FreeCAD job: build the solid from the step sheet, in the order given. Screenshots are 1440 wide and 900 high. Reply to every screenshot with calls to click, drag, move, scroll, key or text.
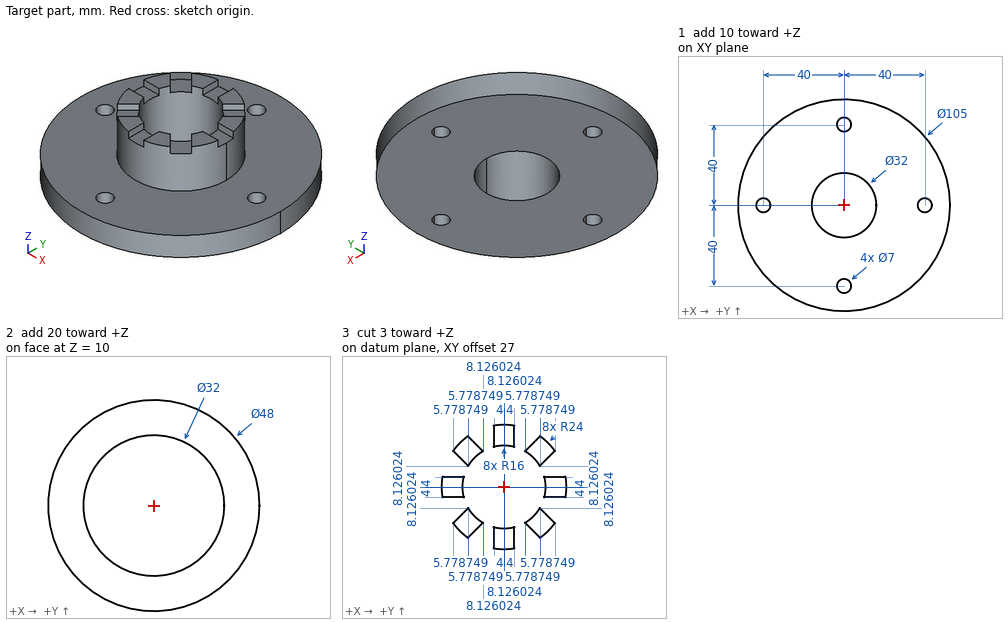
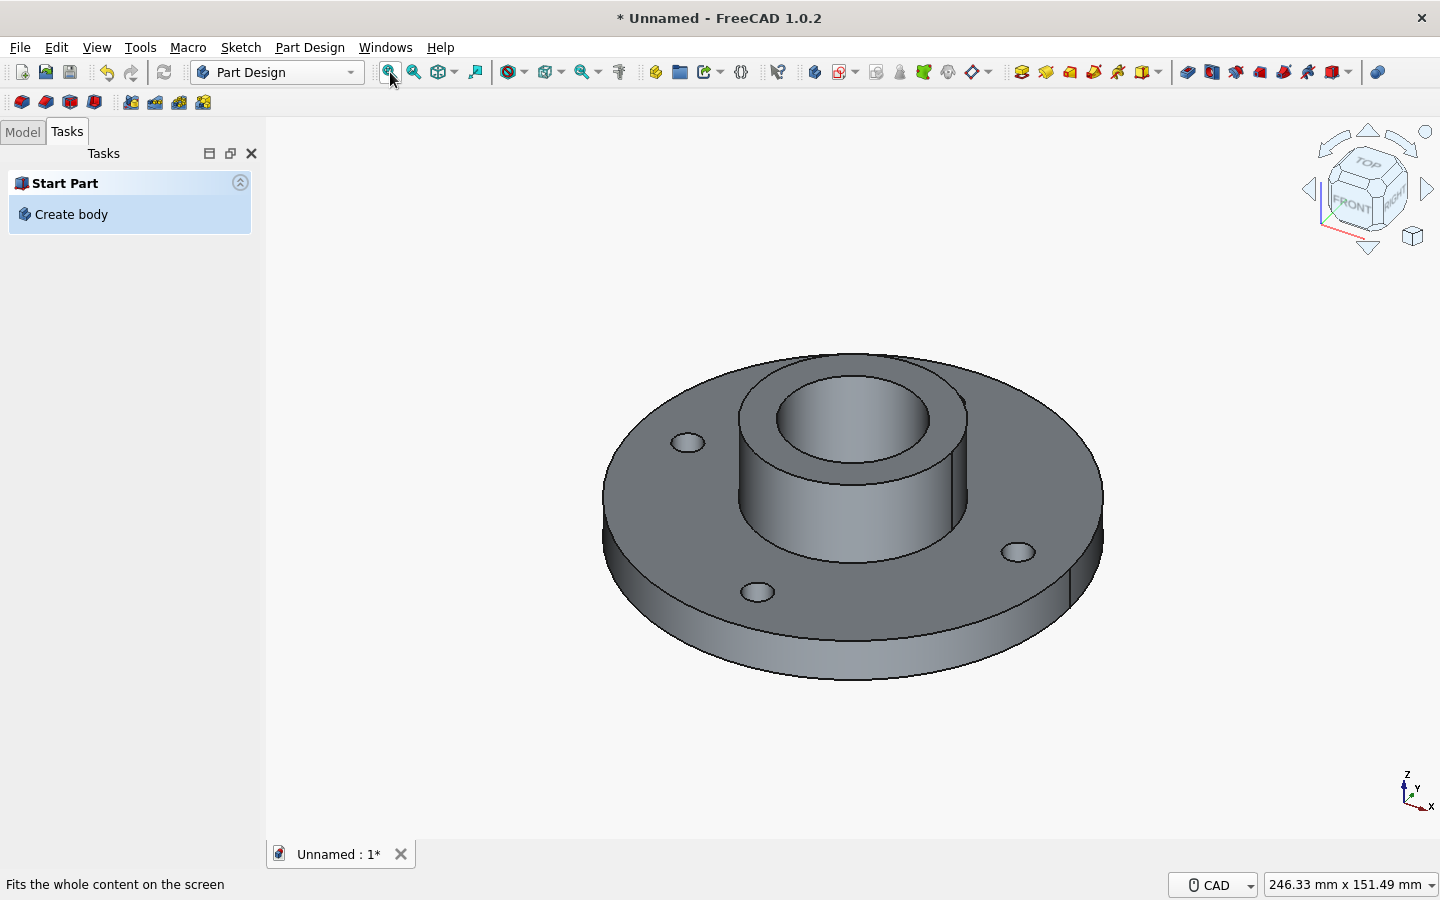
click(23, 131)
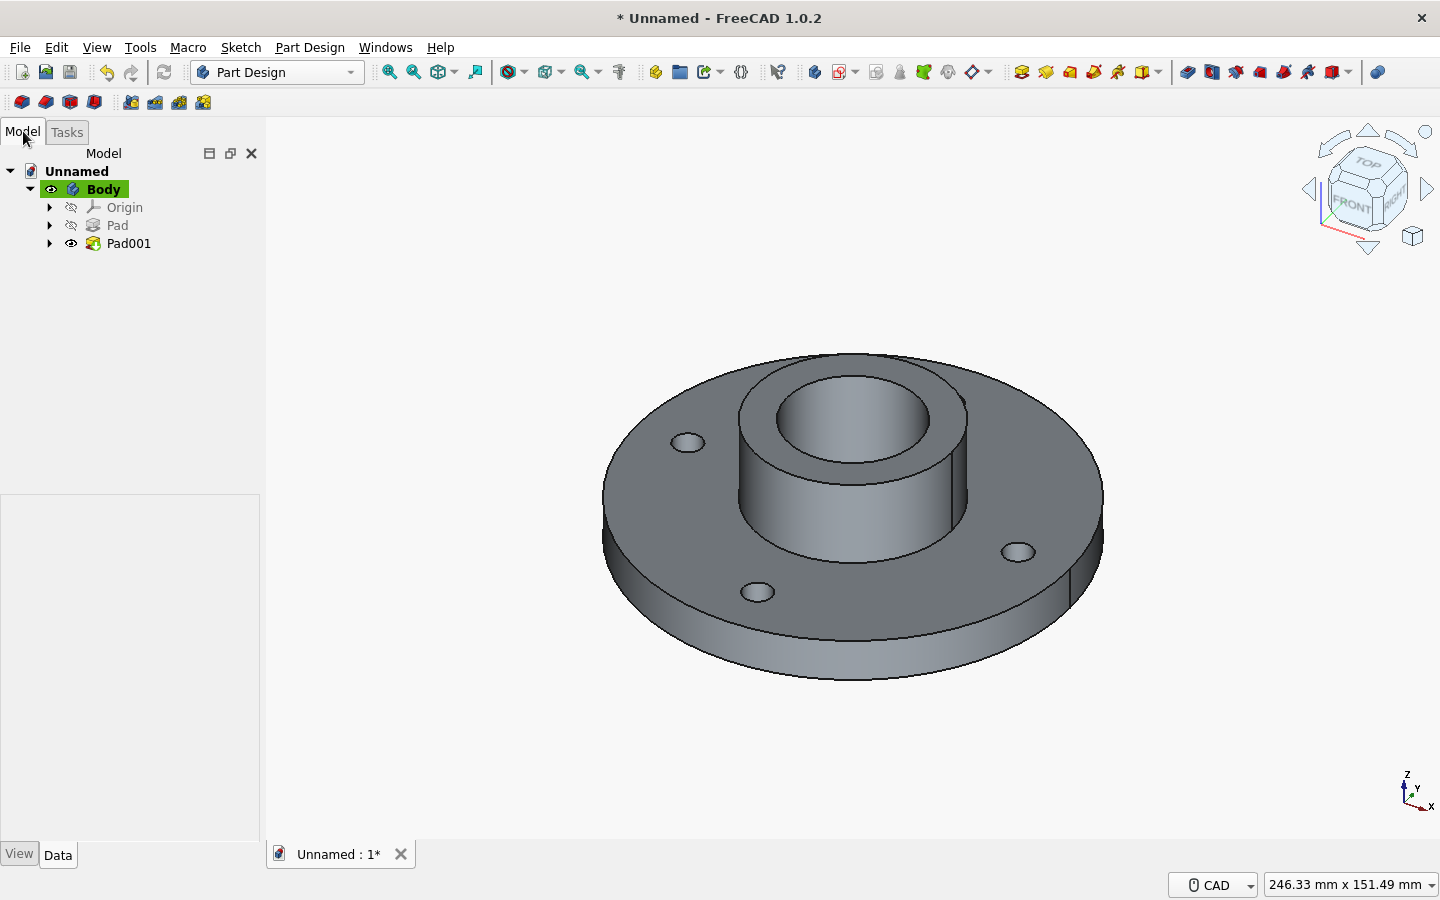
click(50, 207)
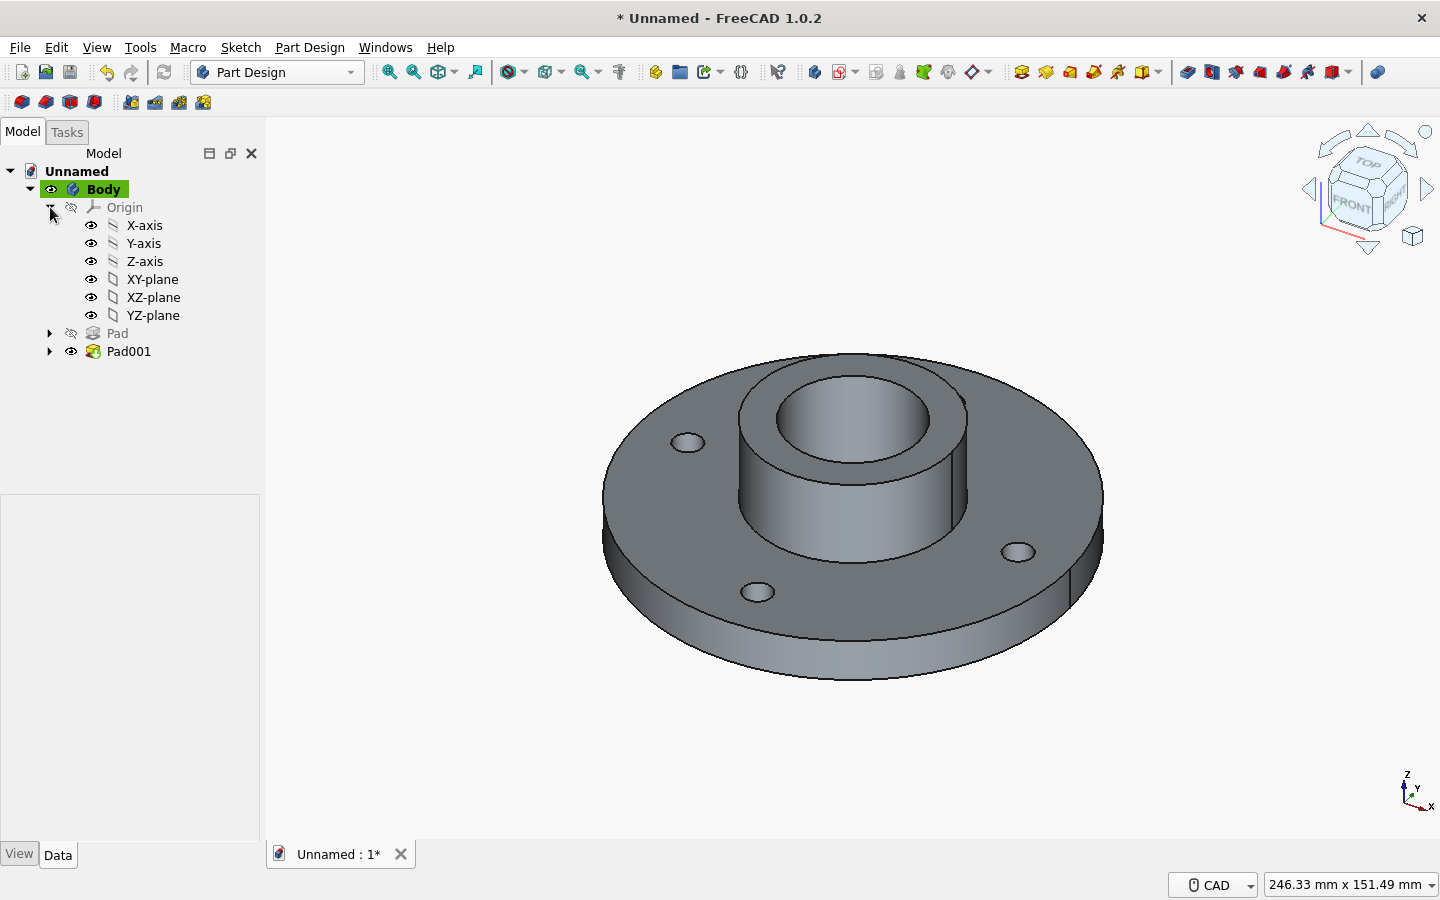
click(136, 279)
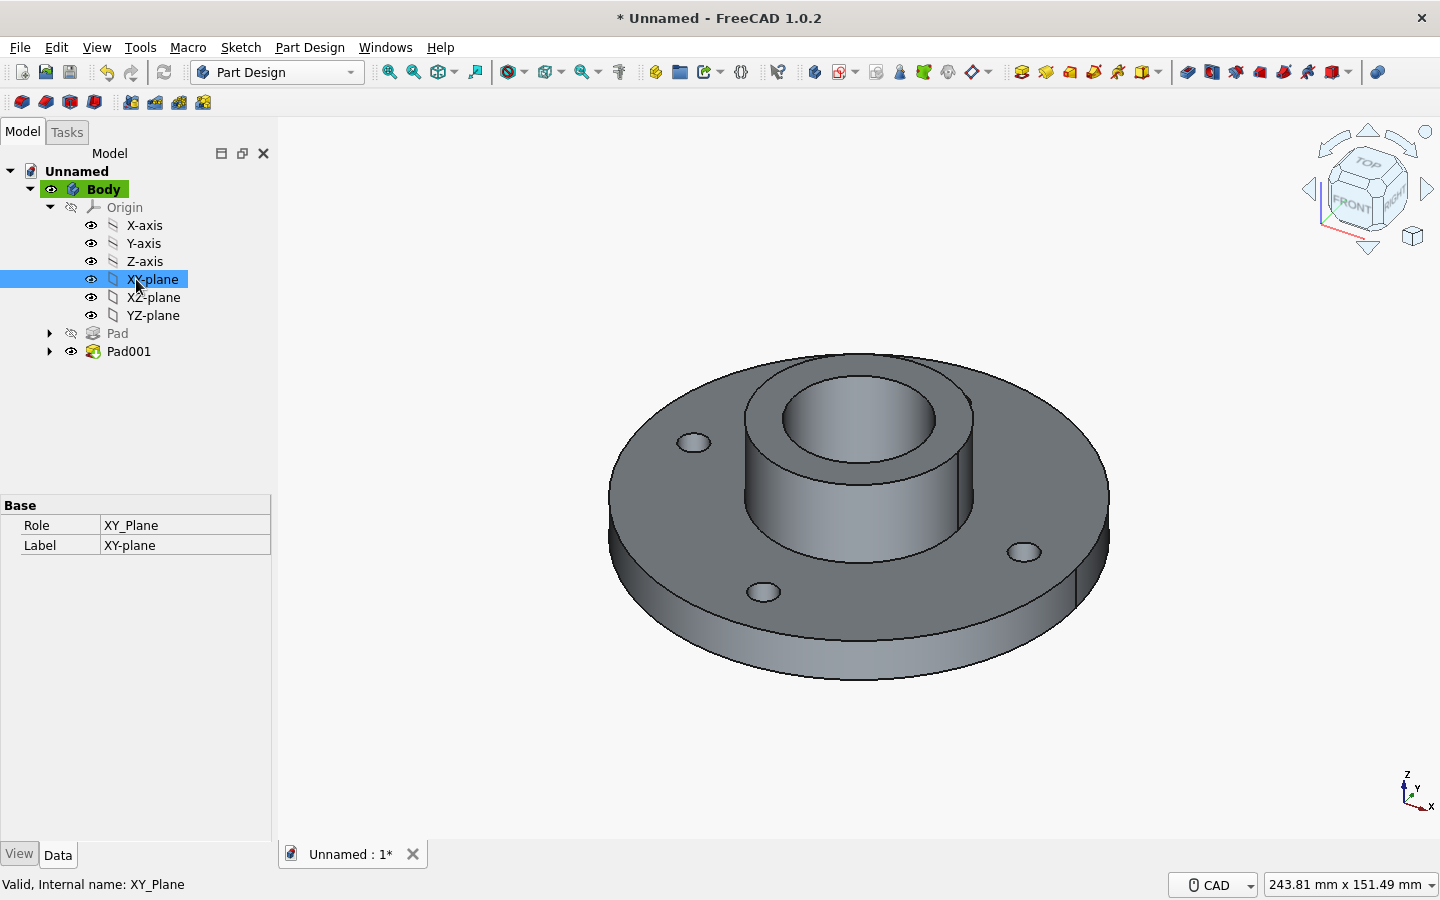
click(972, 72)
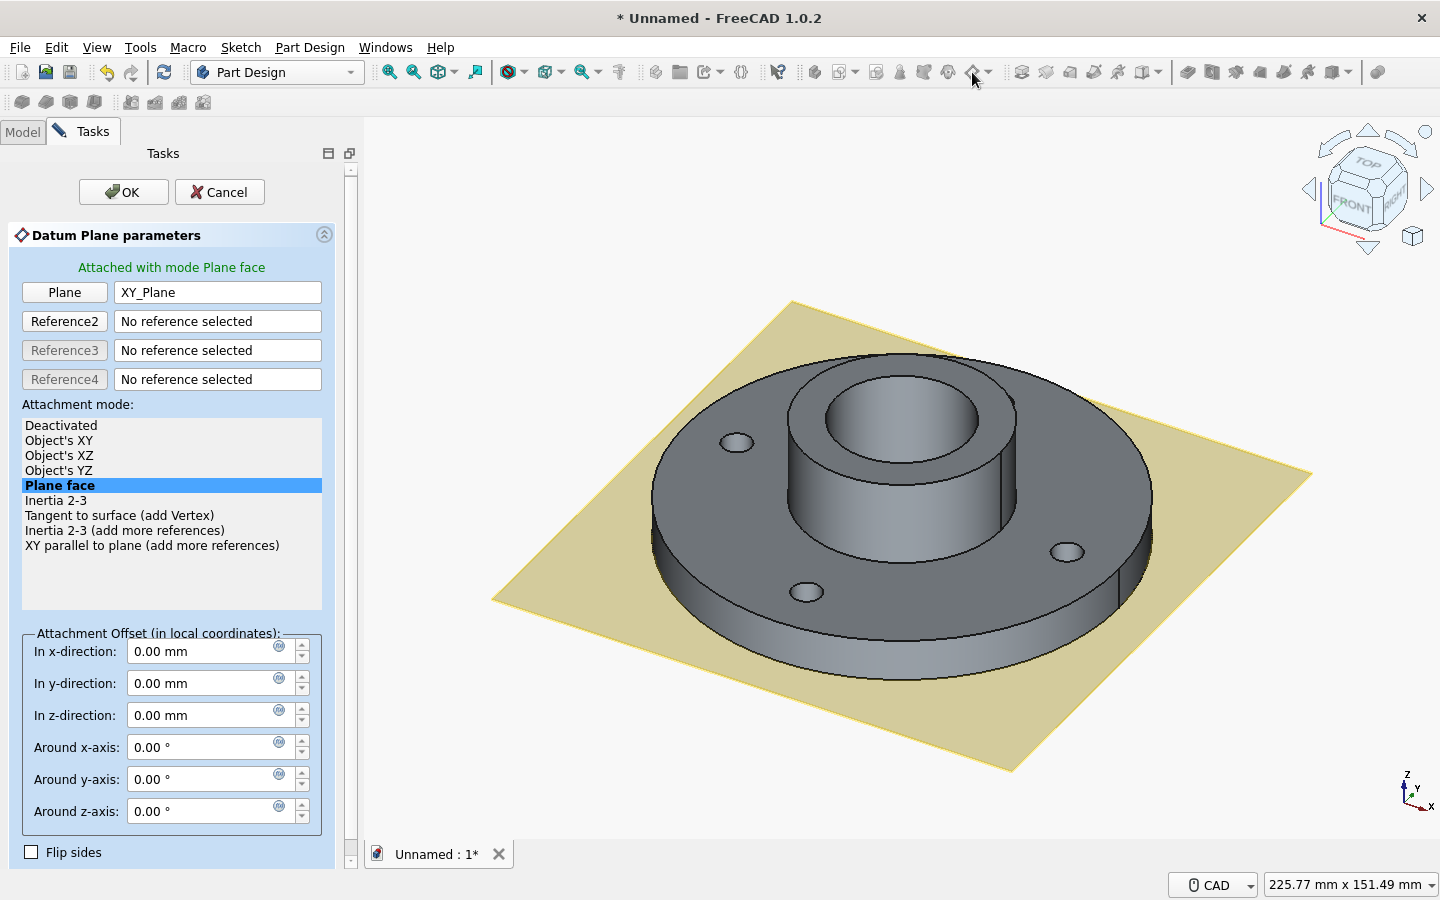
triple_click(210, 715)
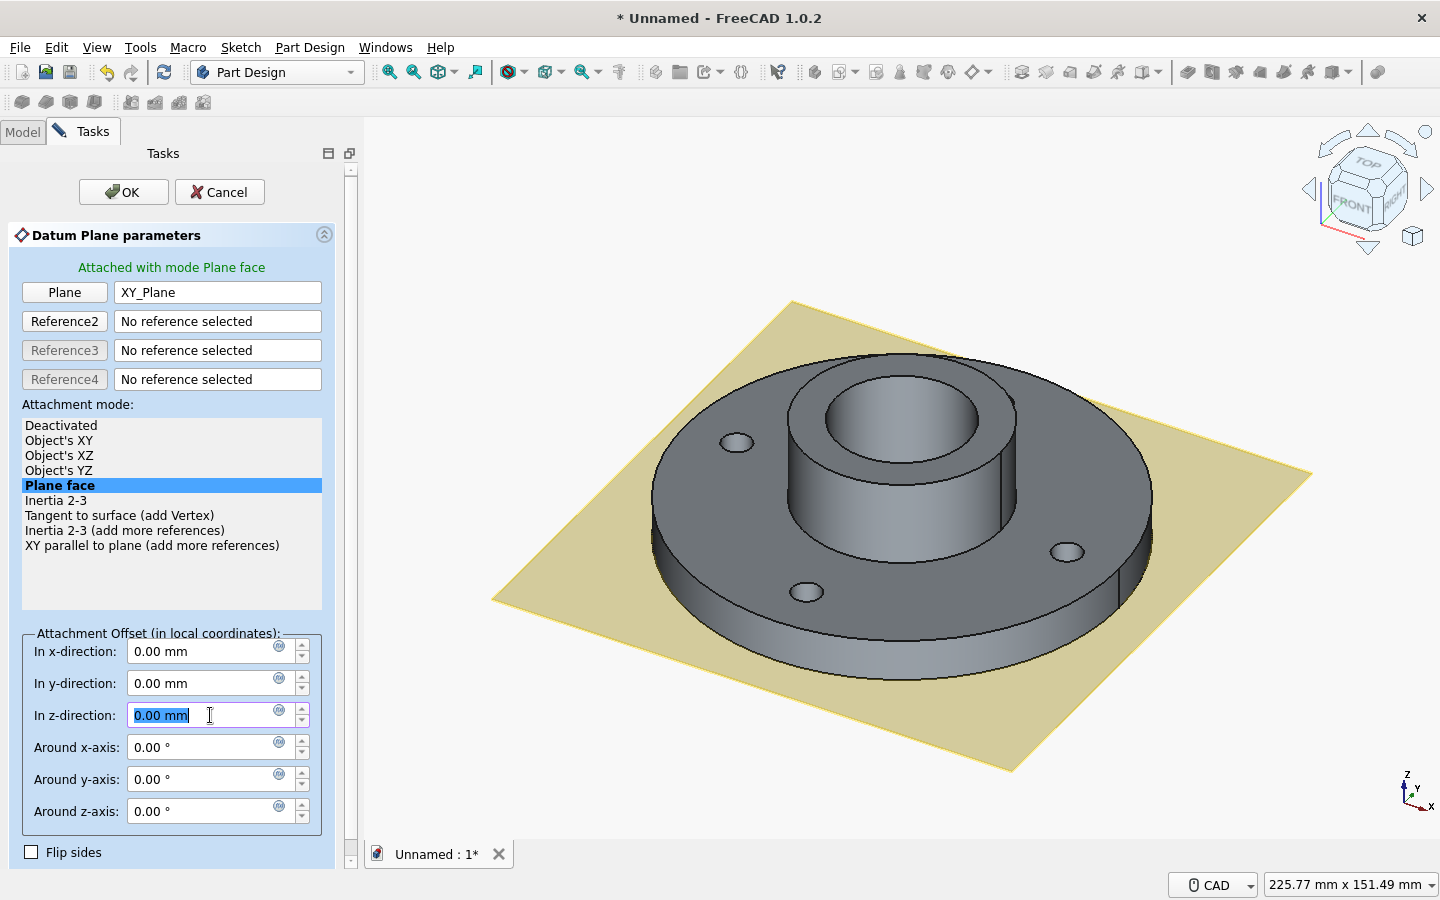
text(27)
key(Tab)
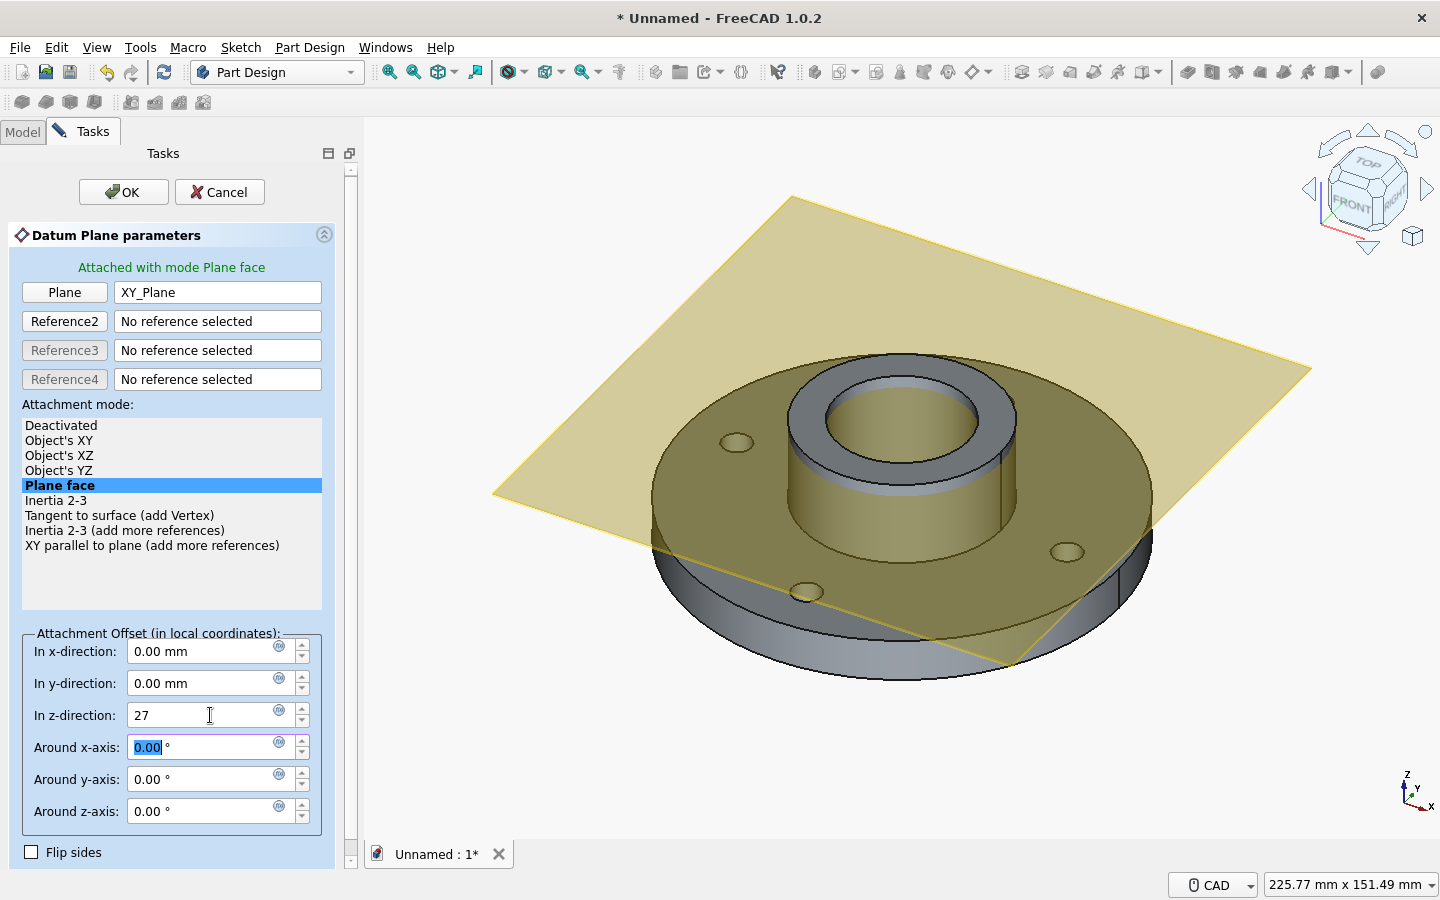
click(124, 192)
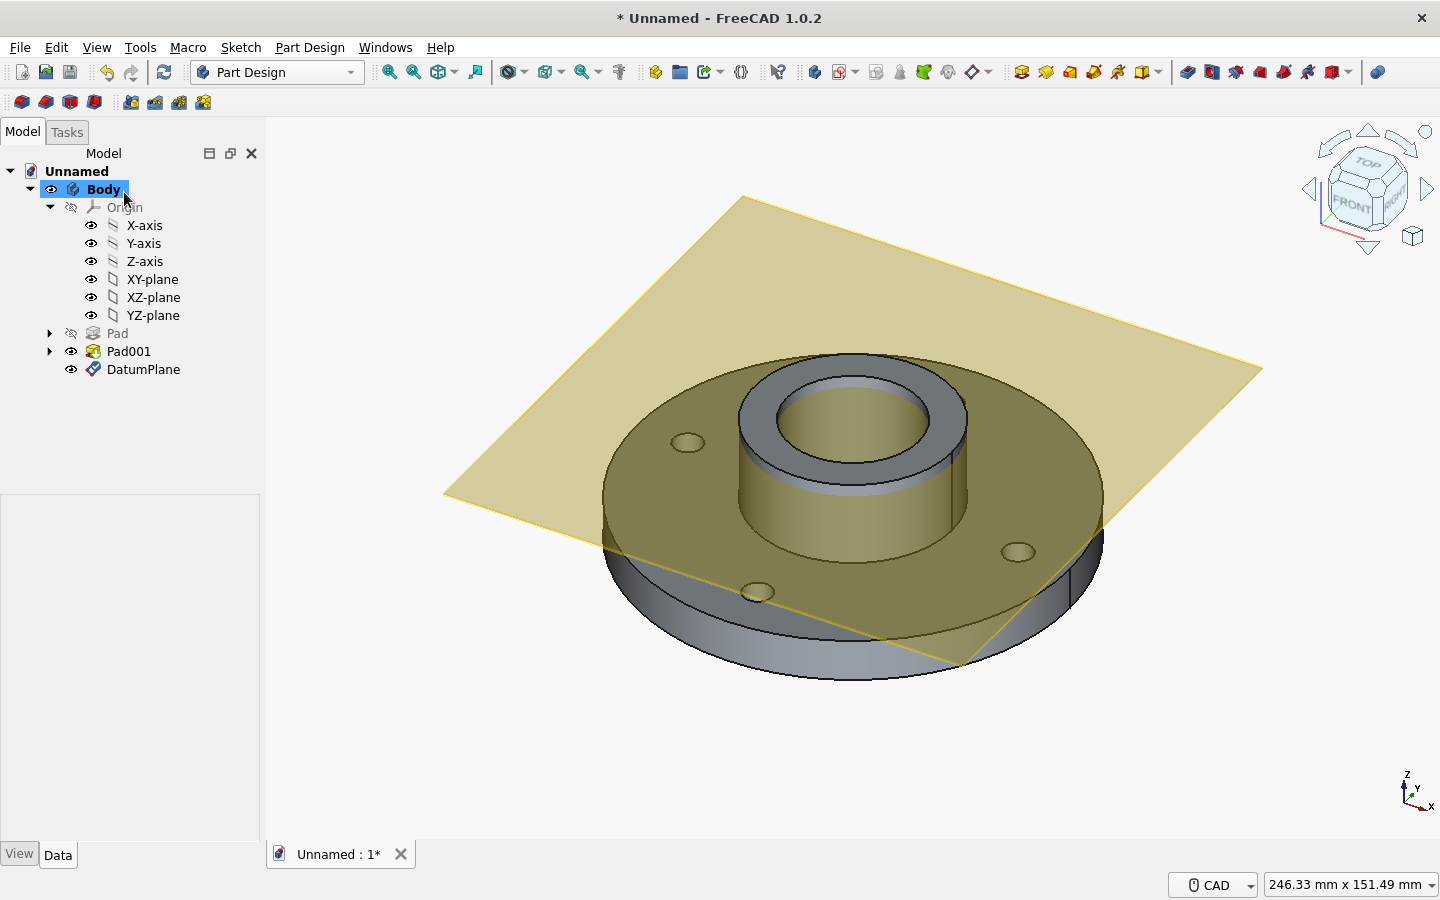
click(116, 369)